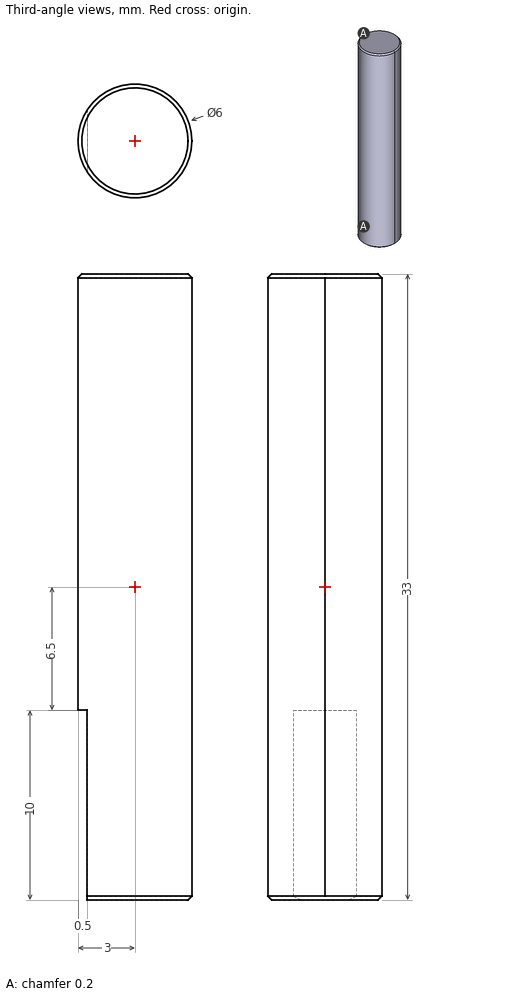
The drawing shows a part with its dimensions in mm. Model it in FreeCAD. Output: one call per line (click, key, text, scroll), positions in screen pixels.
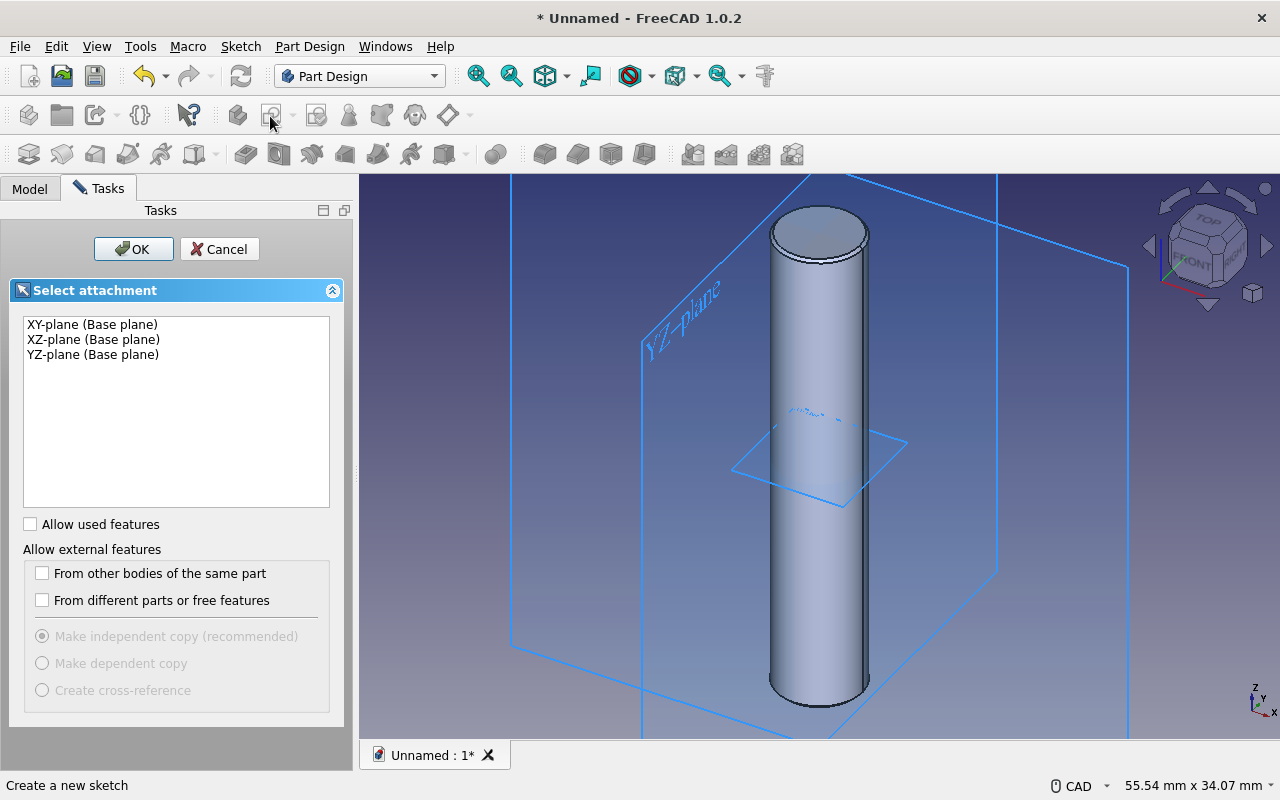
click(84, 340)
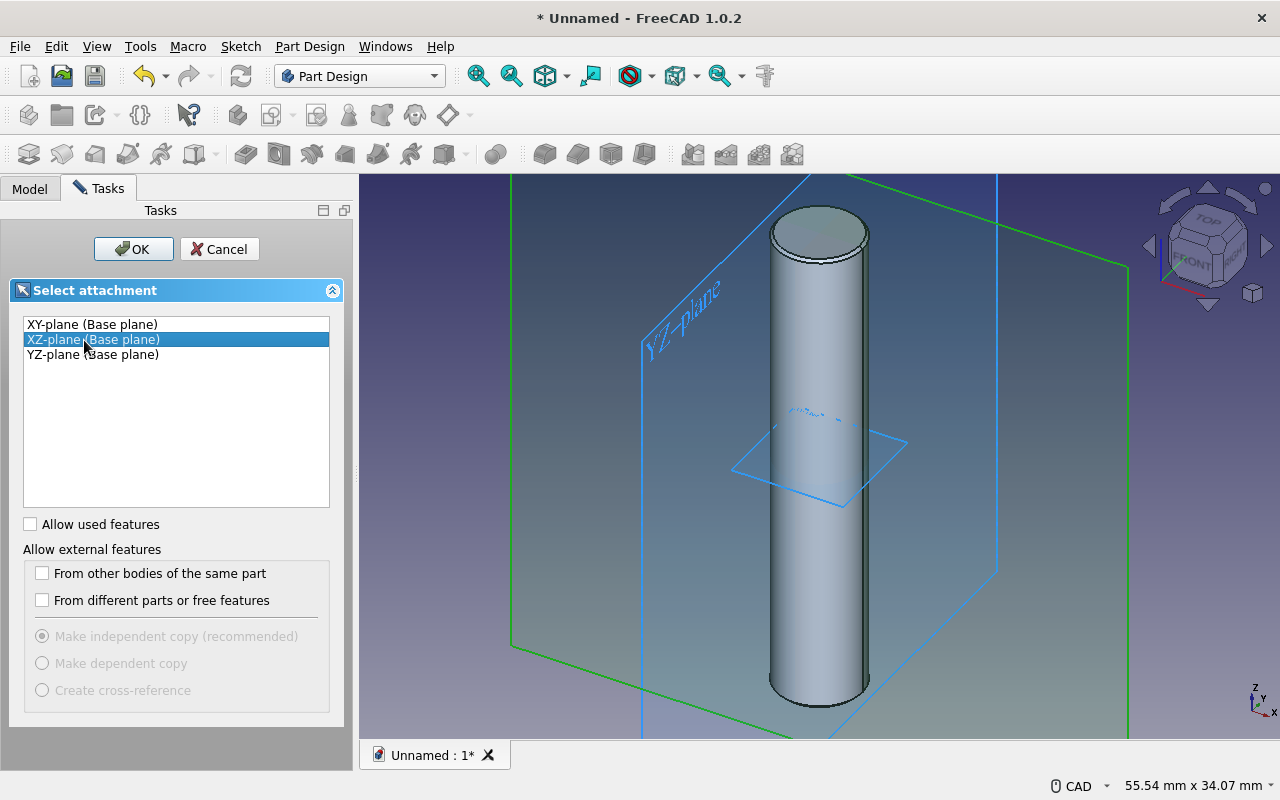
click(134, 249)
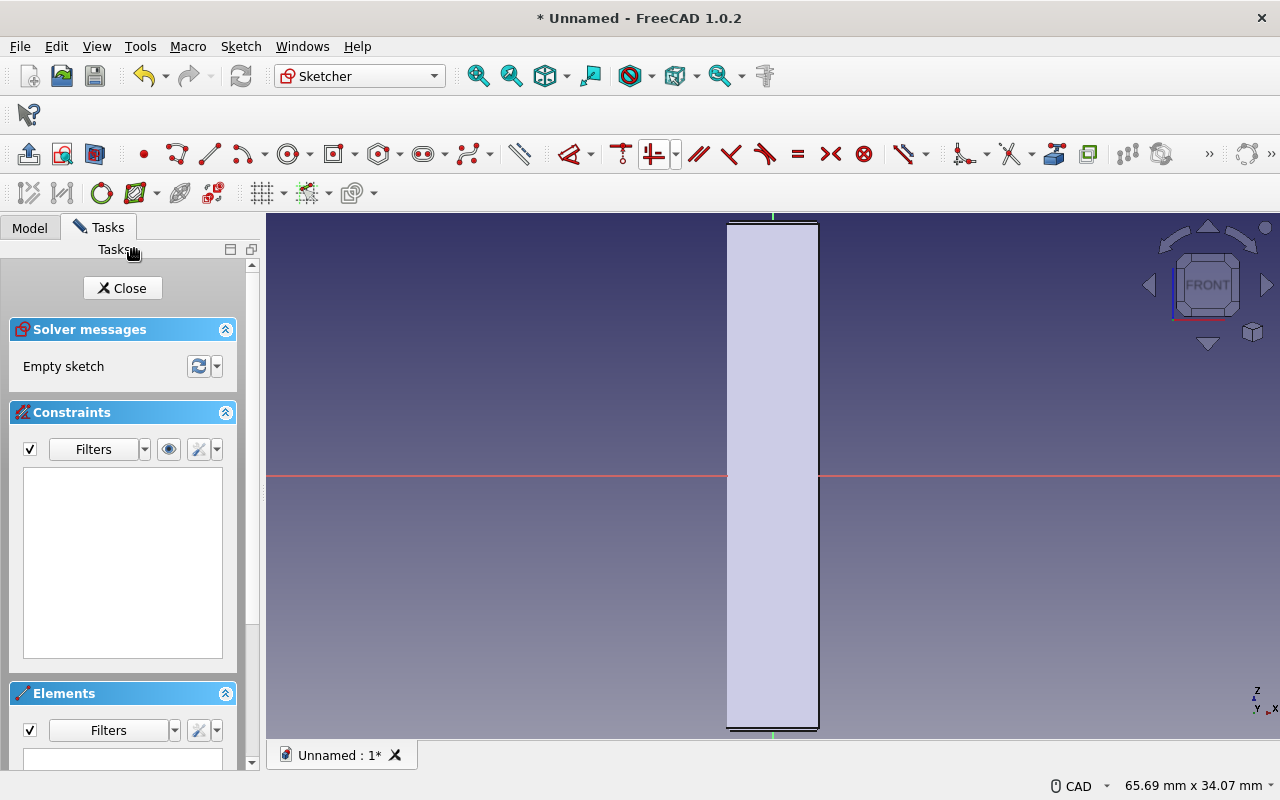
click(95, 154)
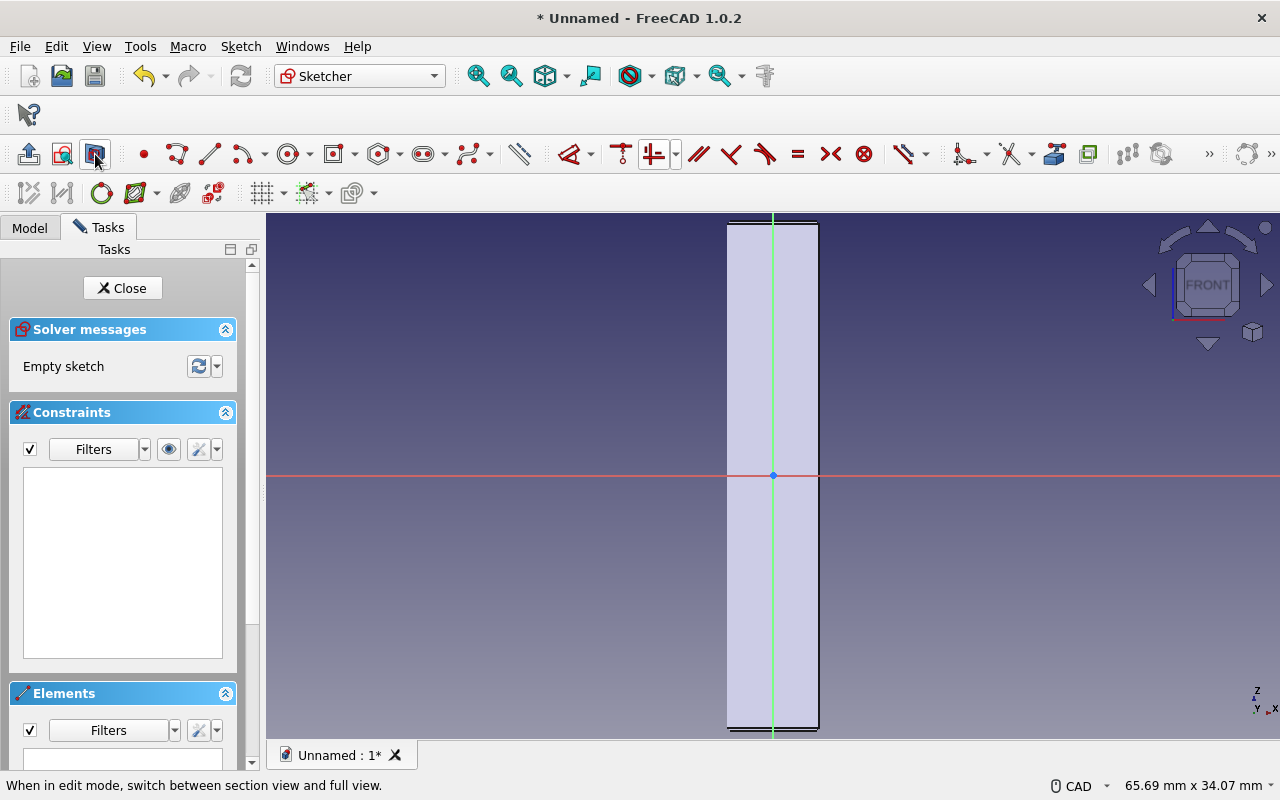
scroll(500, 241, down, 1)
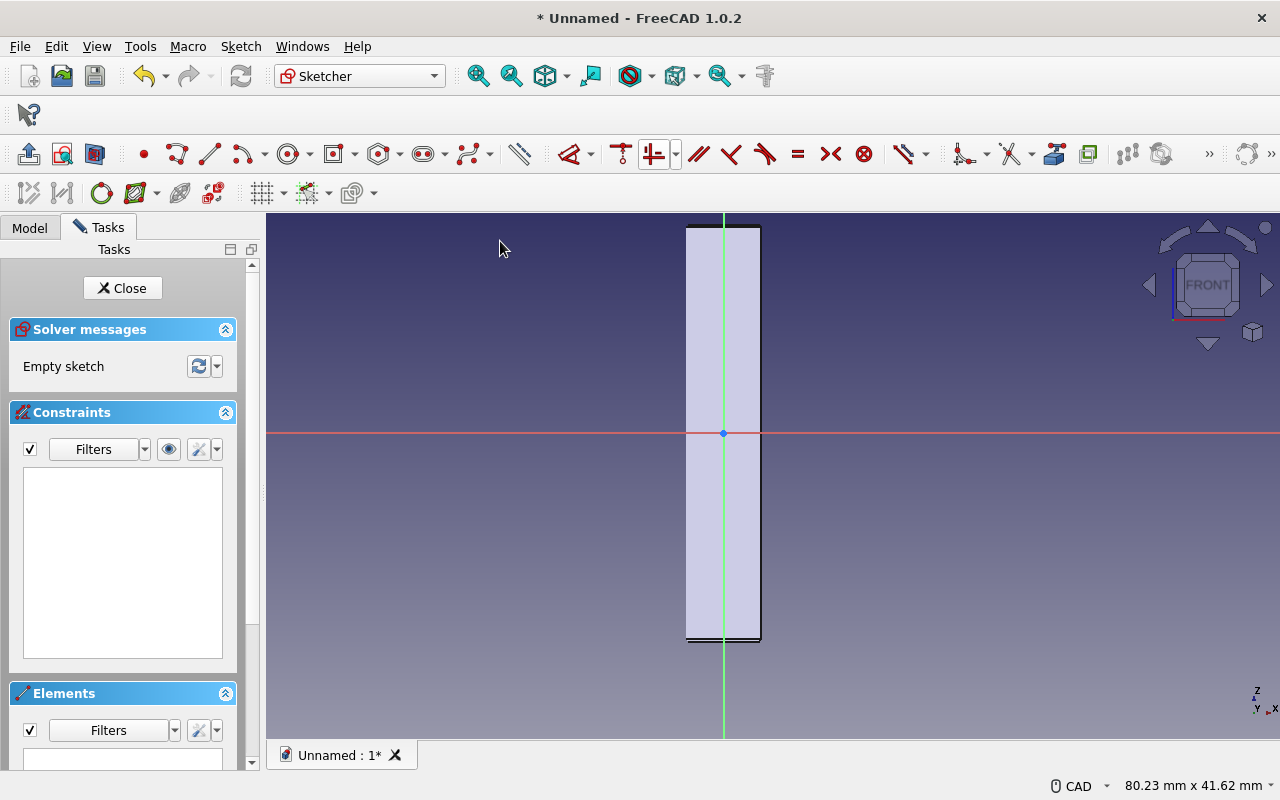
scroll(705, 663, up, 2)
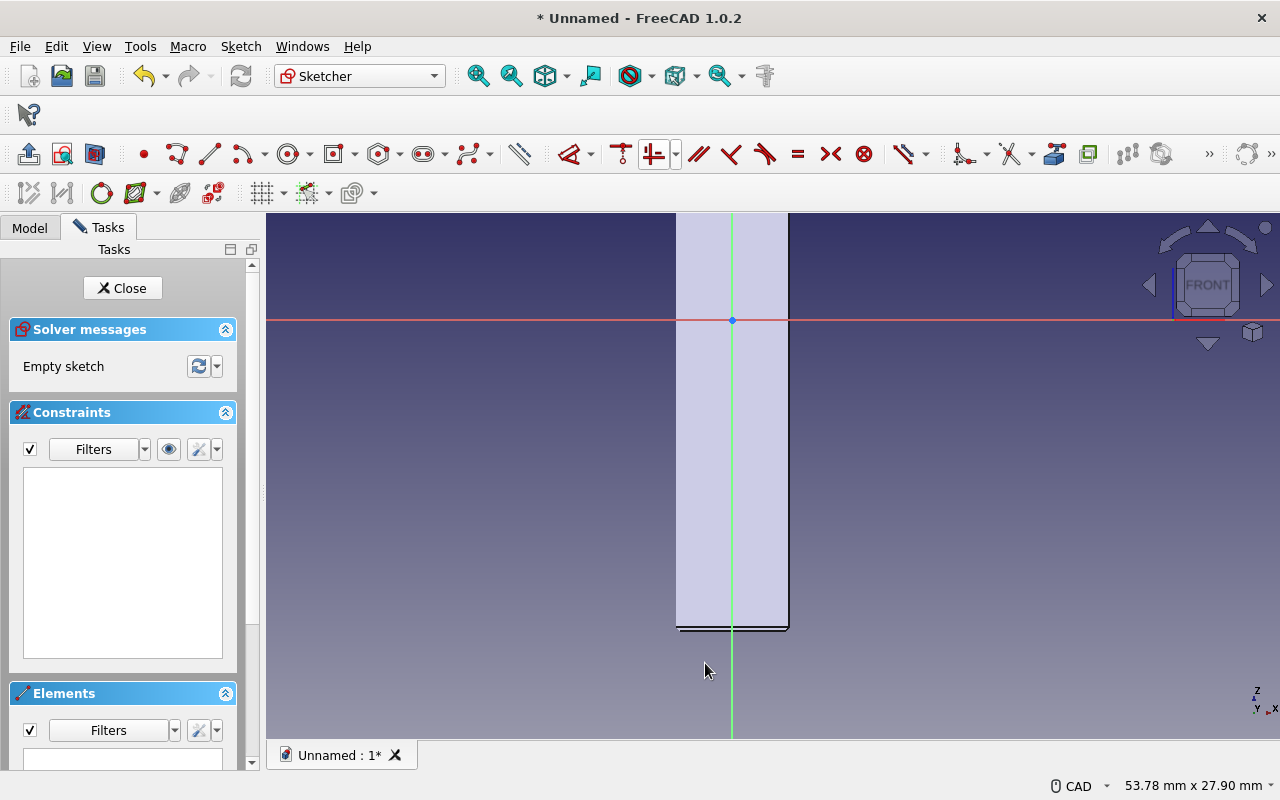
key(g)
key(r)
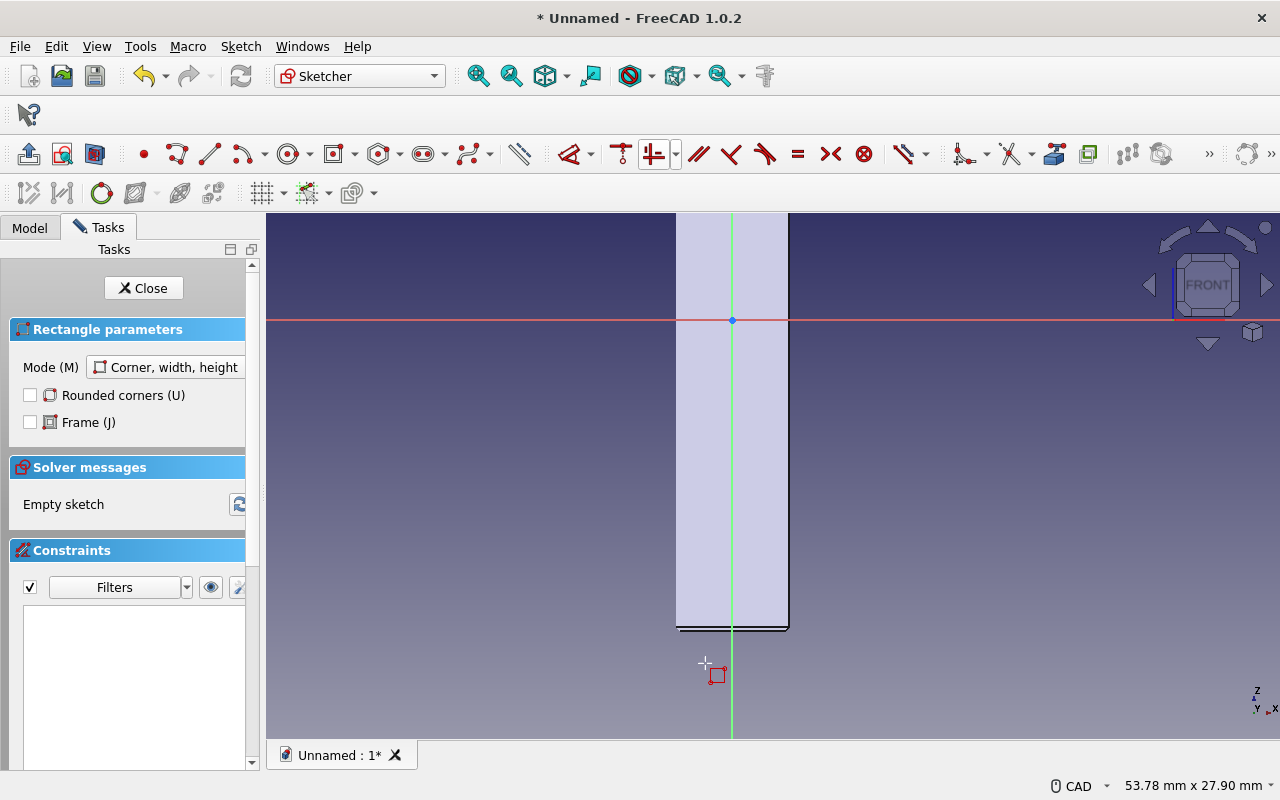
scroll(676, 443, up, 3)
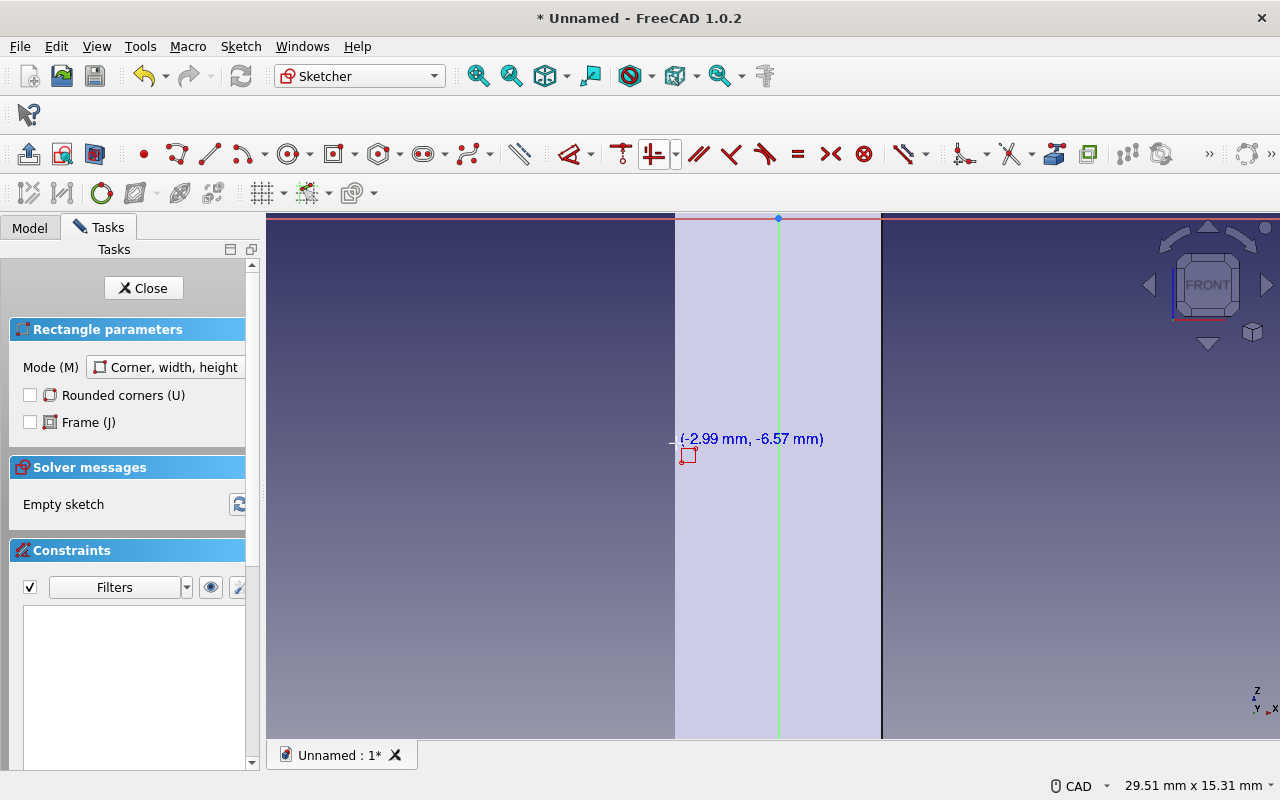
click(675, 442)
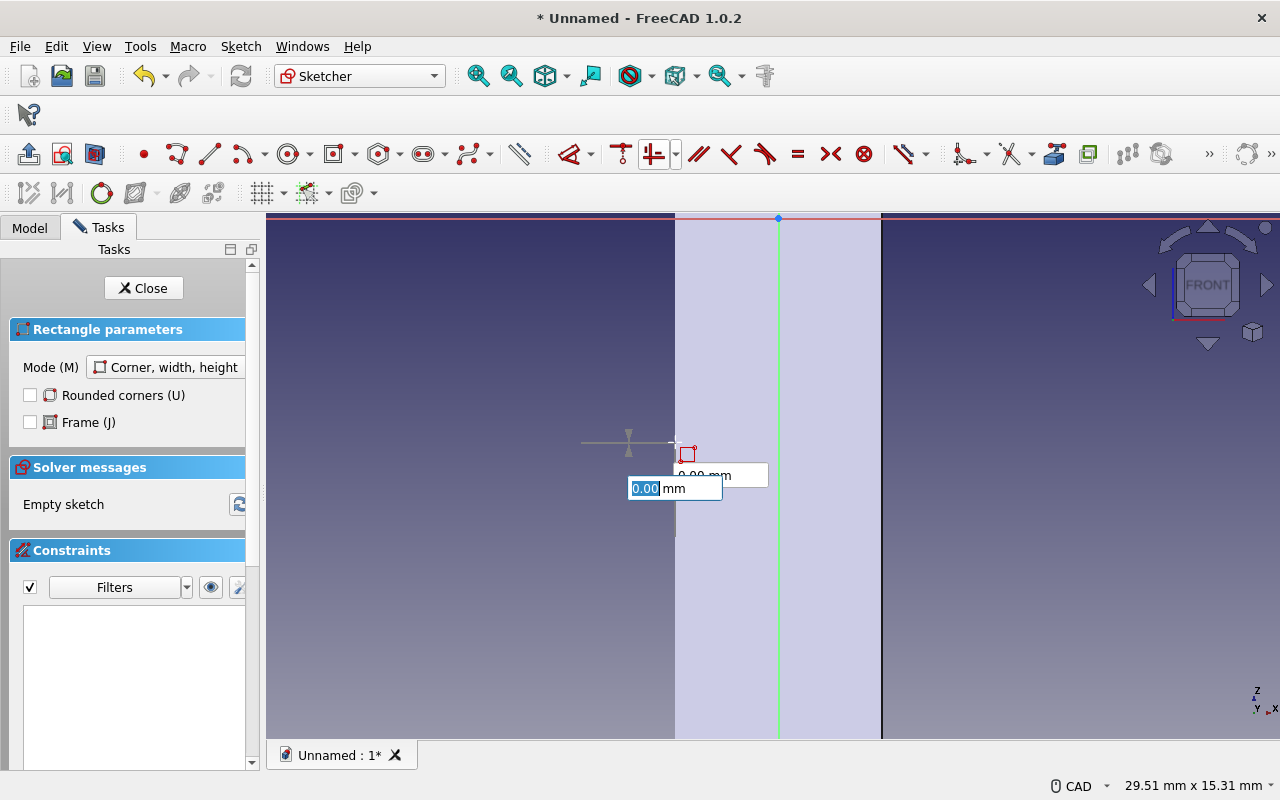
scroll(677, 444, down, 3)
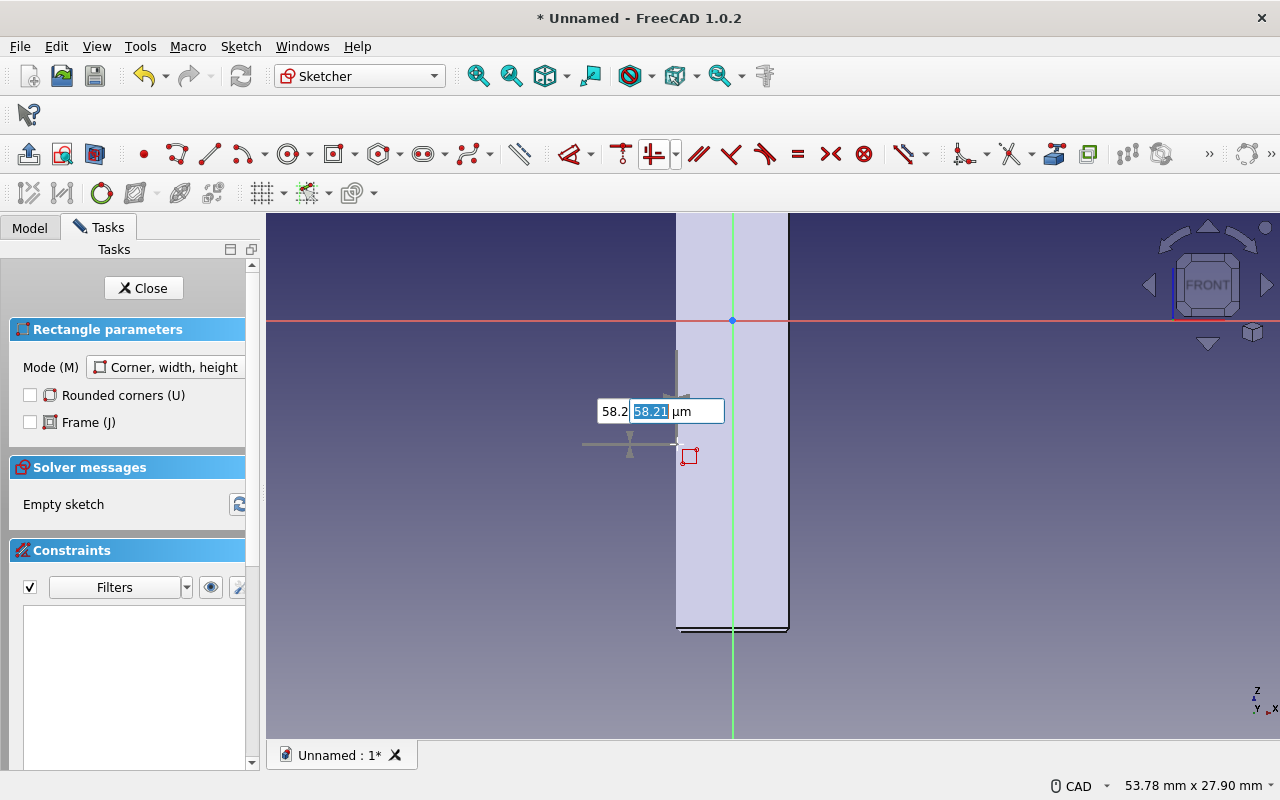
click(686, 632)
key(Escape)